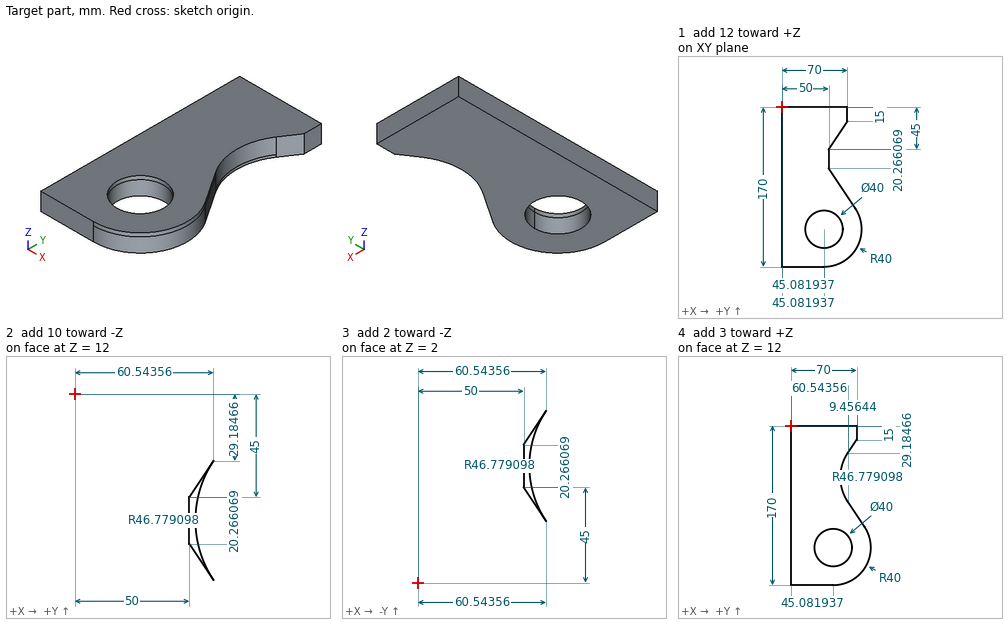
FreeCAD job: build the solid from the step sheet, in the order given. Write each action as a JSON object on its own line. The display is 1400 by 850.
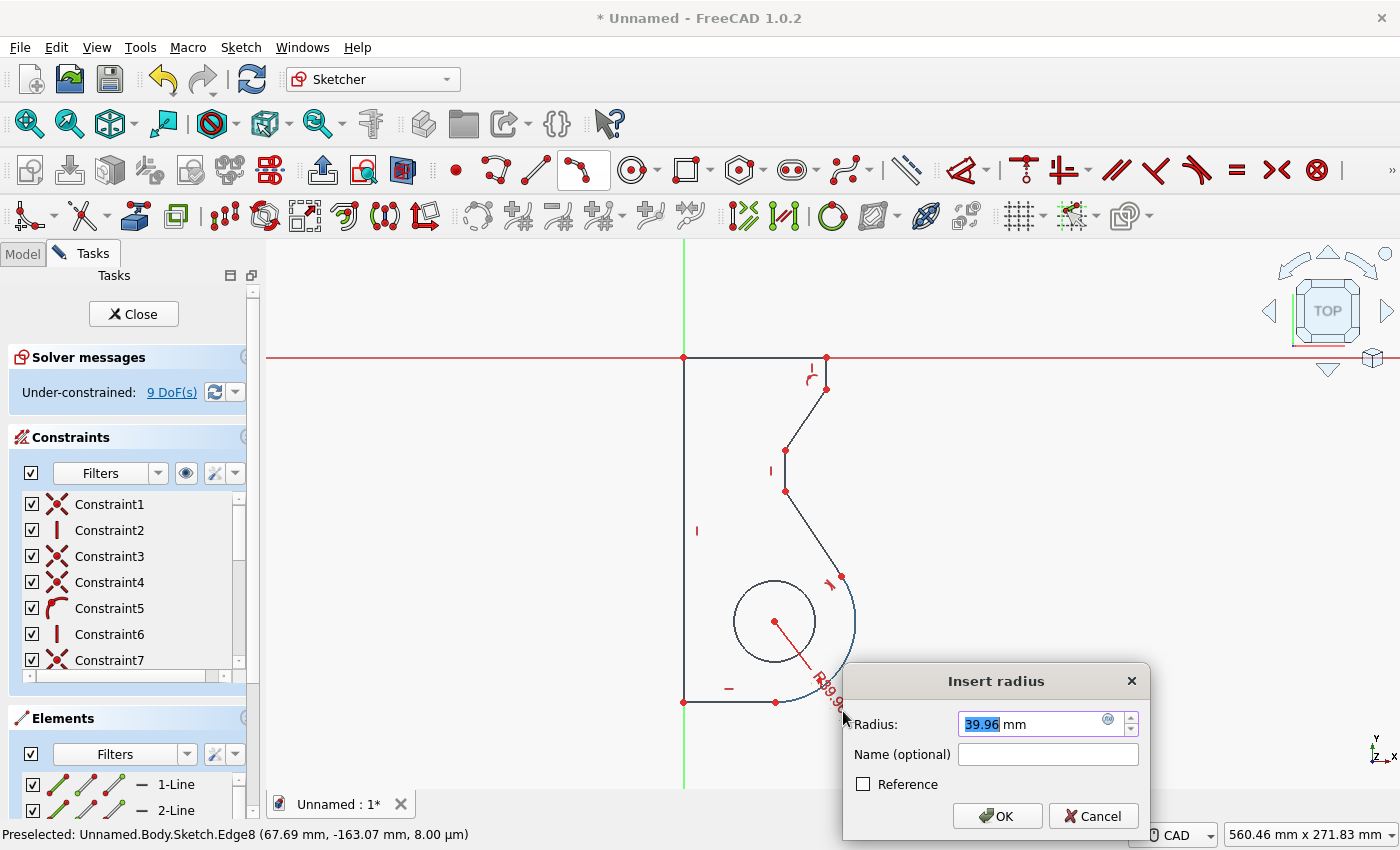
{"action": "type", "text": "40"}
{"action": "key", "text": "Return"}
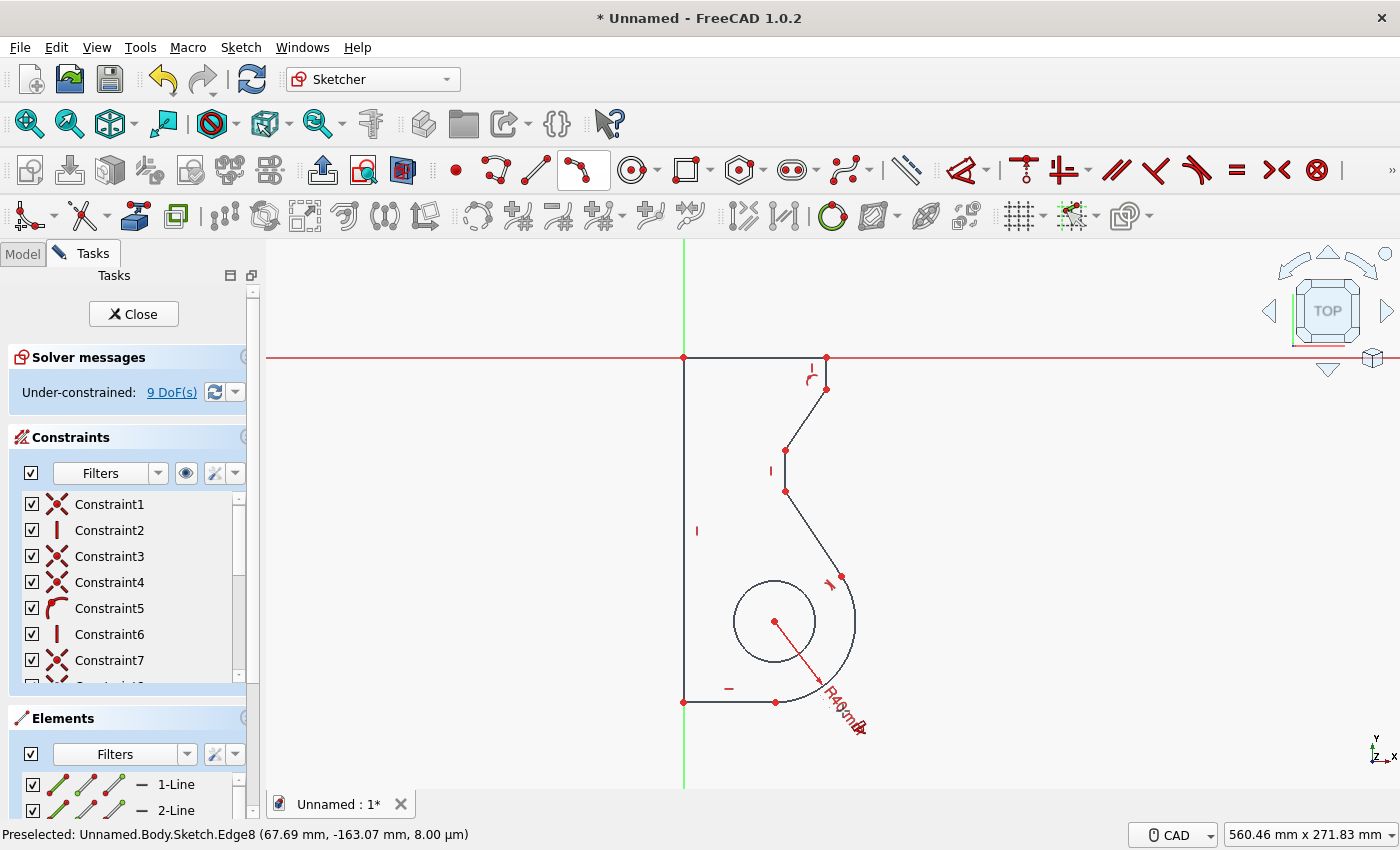
{"action": "left_click", "coordinate": [803, 593]}
{"action": "left_click", "coordinate": [795, 552]}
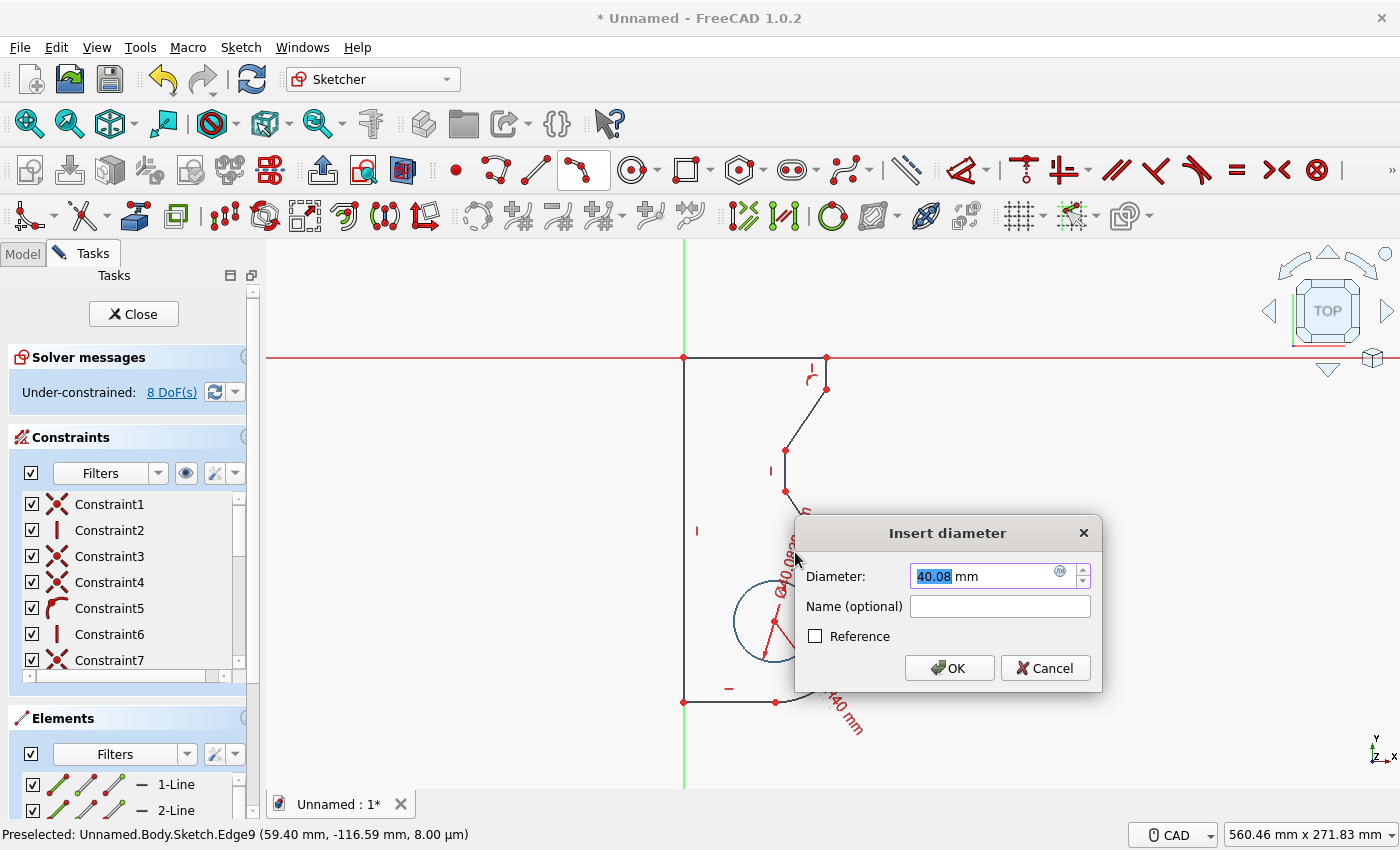
{"action": "type", "text": "40"}
{"action": "key", "text": "Return"}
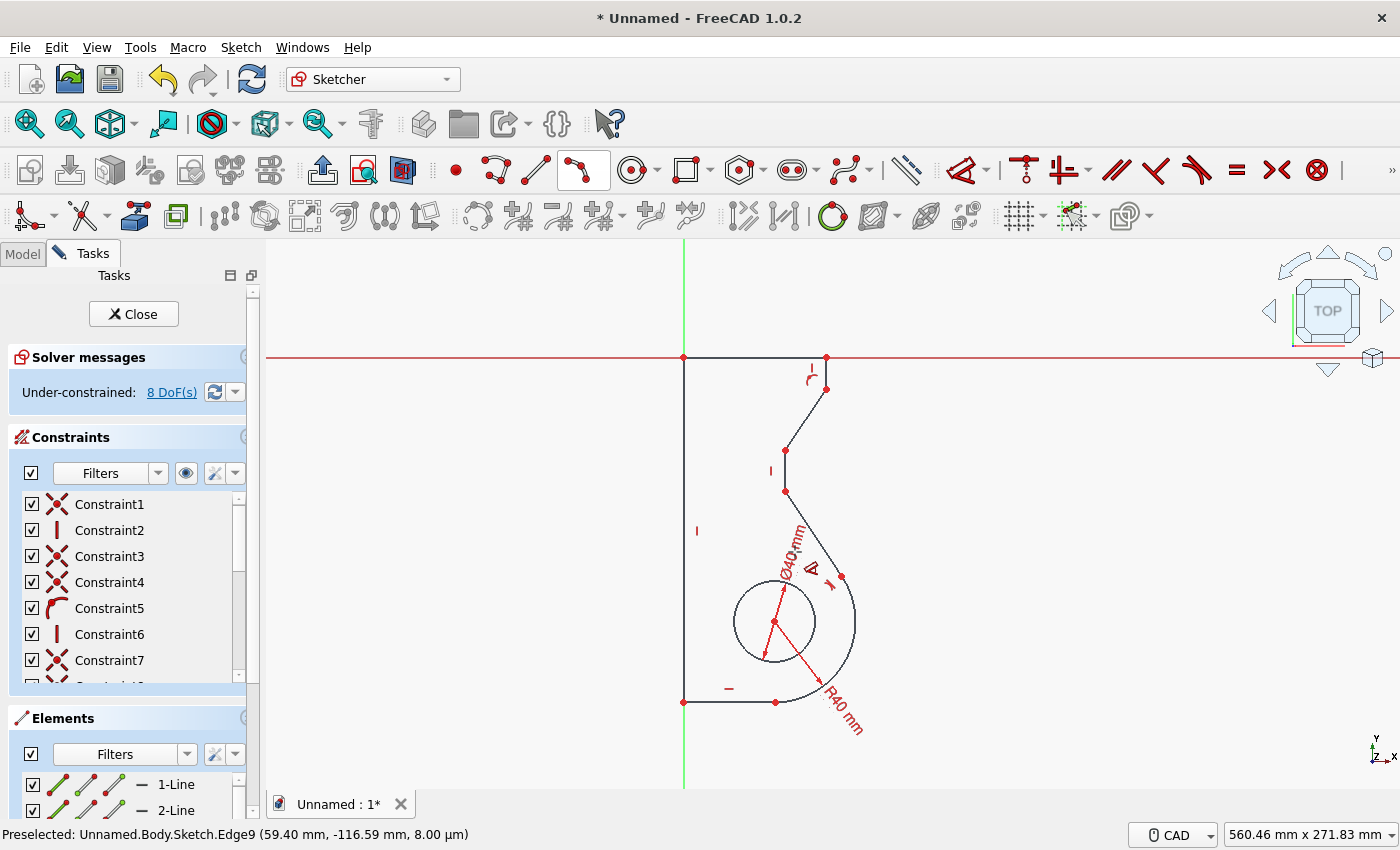
{"action": "scroll", "coordinate": [826, 380], "scroll_direction": "up", "scroll_amount": 2}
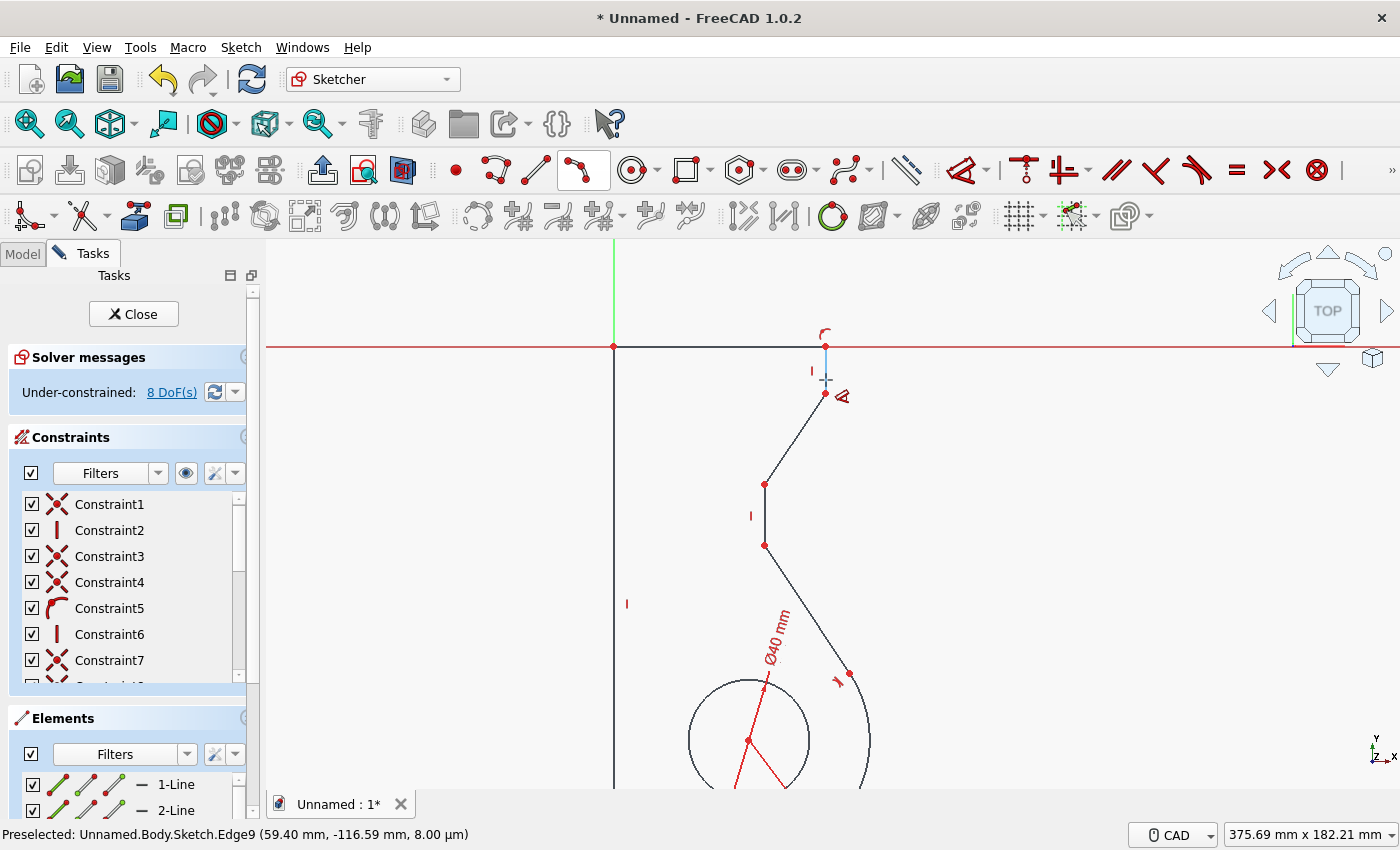
{"action": "left_click", "coordinate": [826, 380]}
{"action": "left_click", "coordinate": [860, 370]}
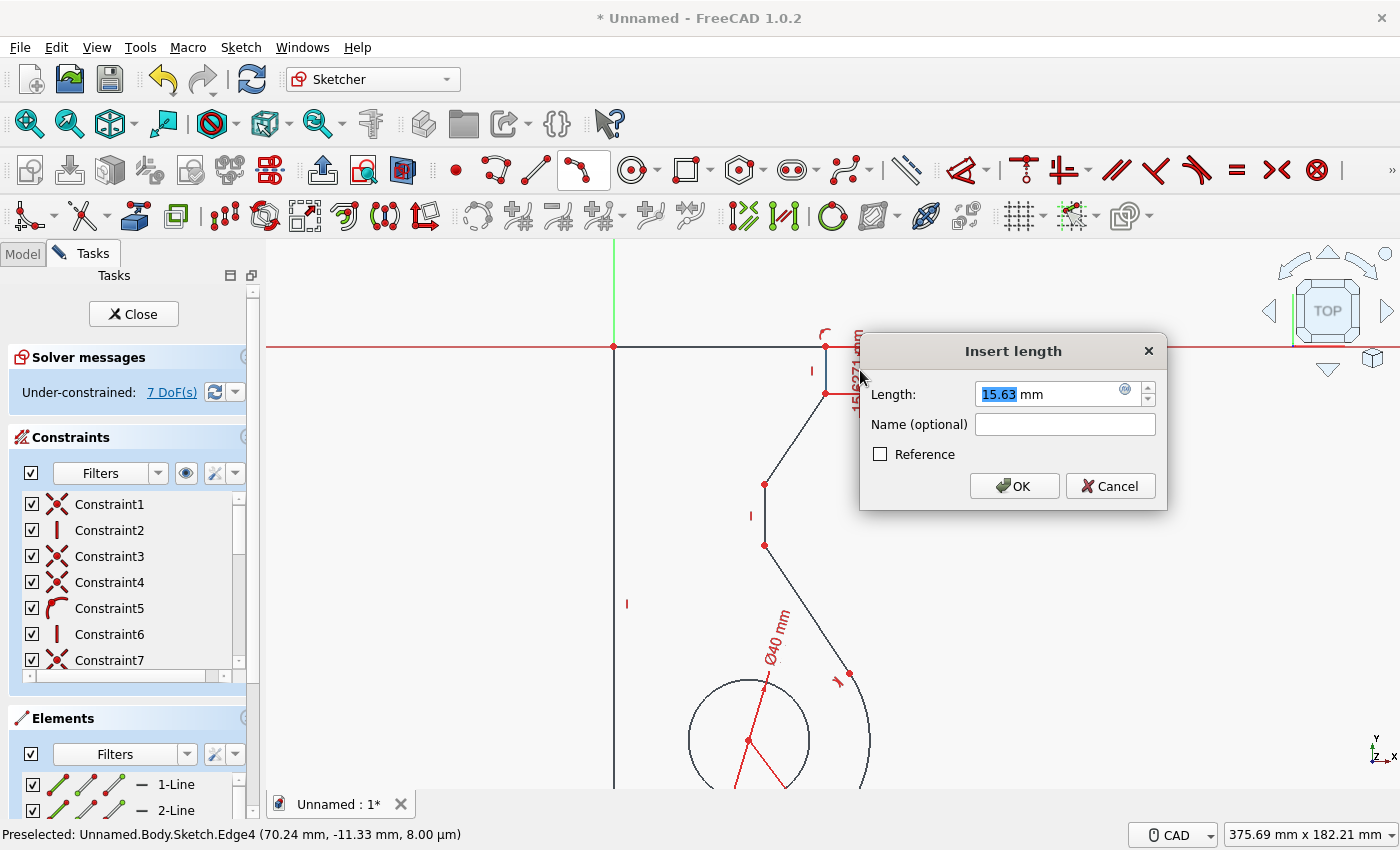
{"action": "type", "text": "15"}
{"action": "key", "text": "Return"}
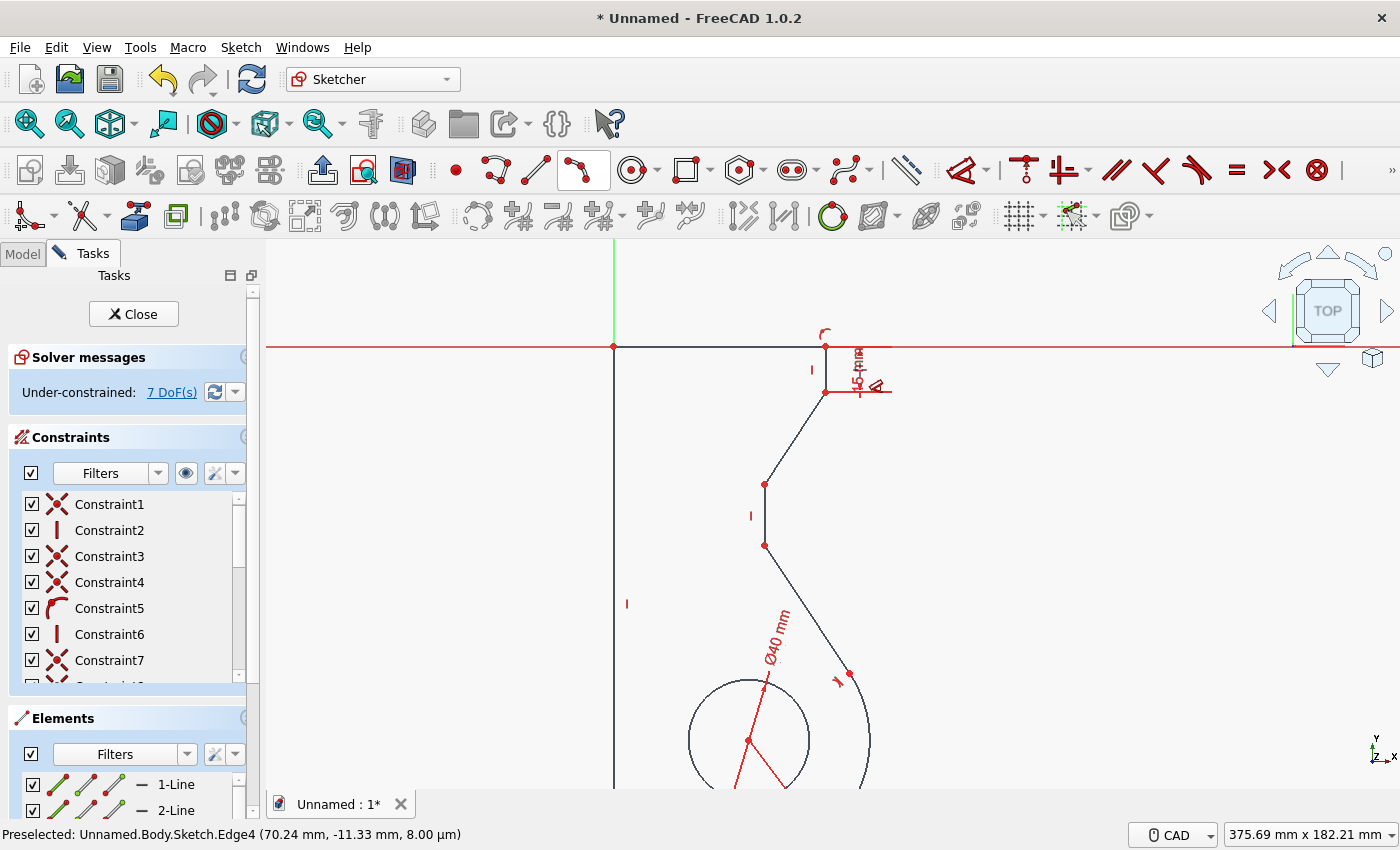
{"action": "left_click", "coordinate": [762, 347]}
{"action": "left_click", "coordinate": [720, 313]}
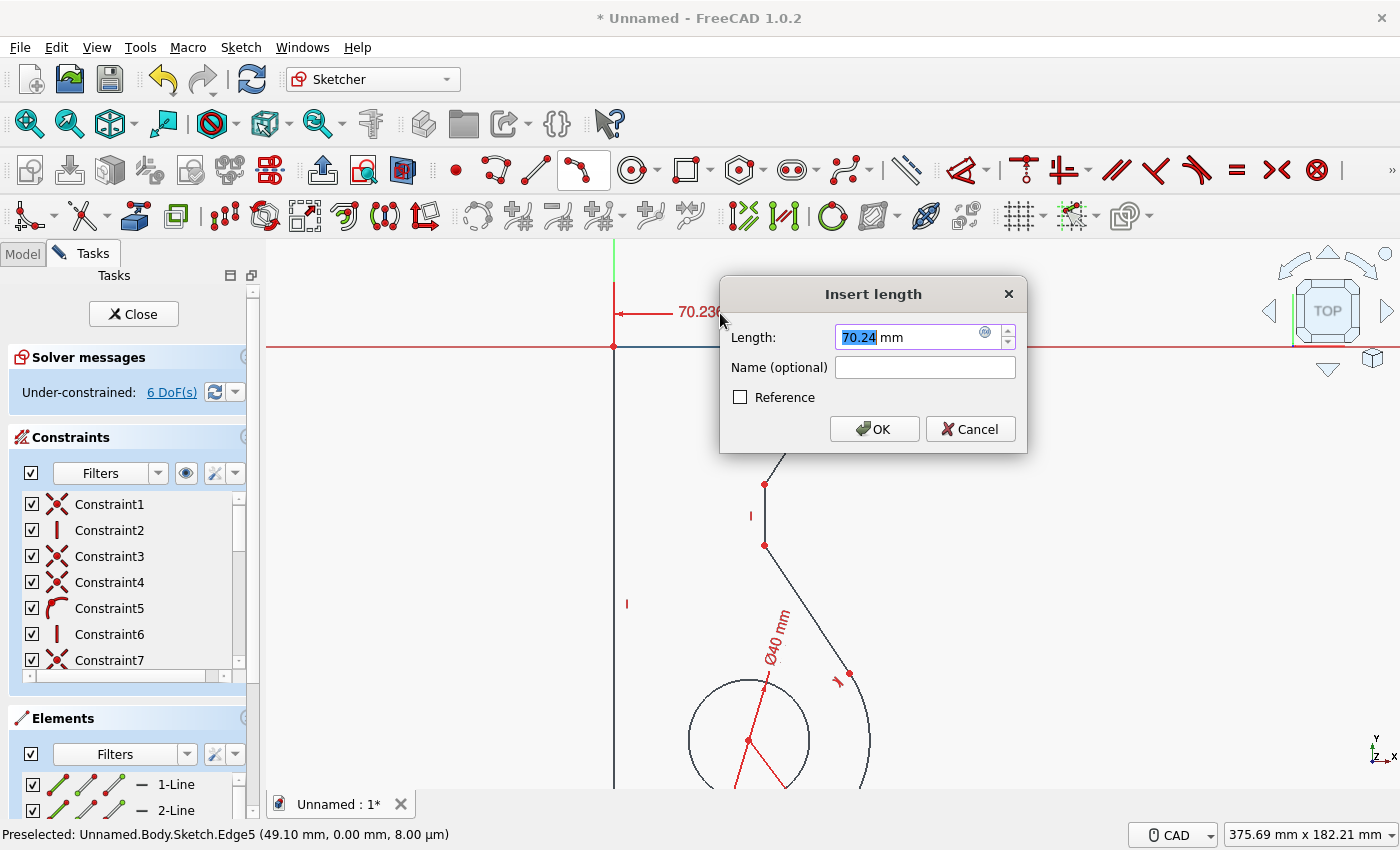
{"action": "type", "text": "70"}
{"action": "key", "text": "Return"}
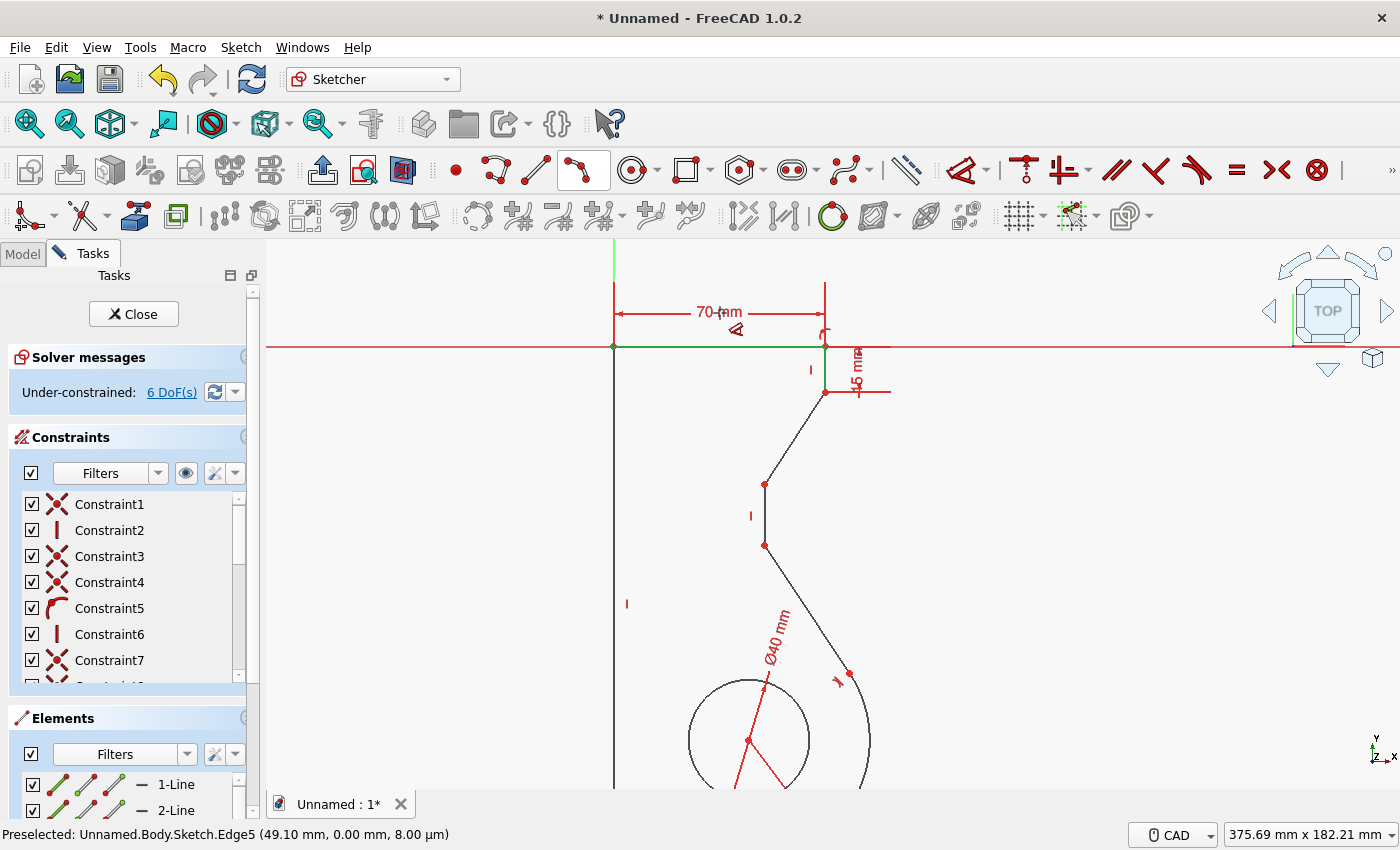
{"action": "left_click", "coordinate": [614, 501]}
{"action": "left_click", "coordinate": [580, 554]}